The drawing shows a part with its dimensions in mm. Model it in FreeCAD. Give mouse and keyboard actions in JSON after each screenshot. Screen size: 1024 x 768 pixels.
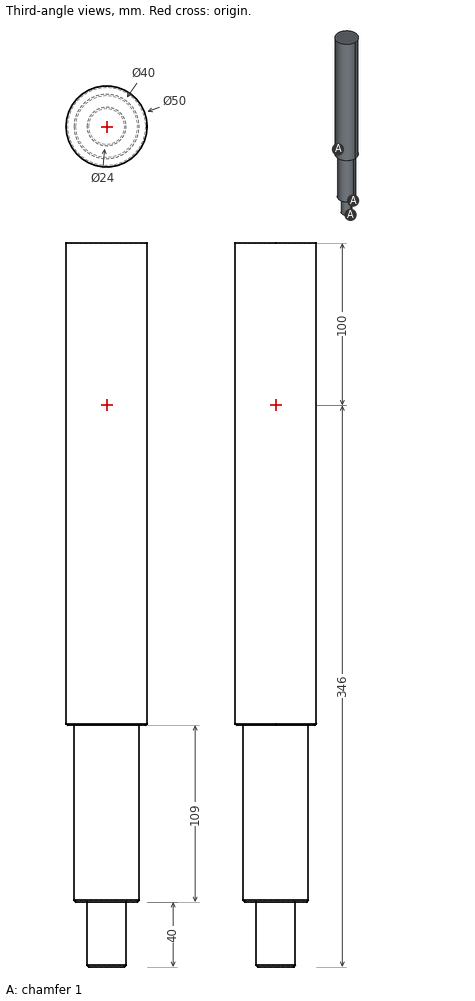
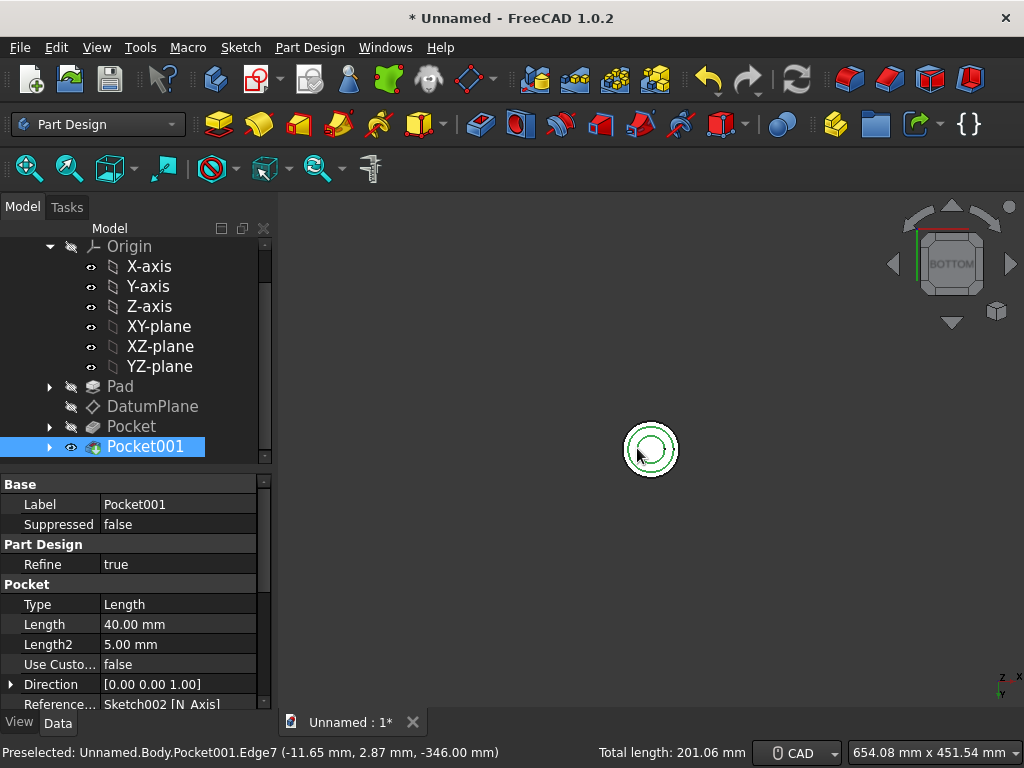
{"action": "left_click", "coordinate": [622, 448], "text": "ctrl"}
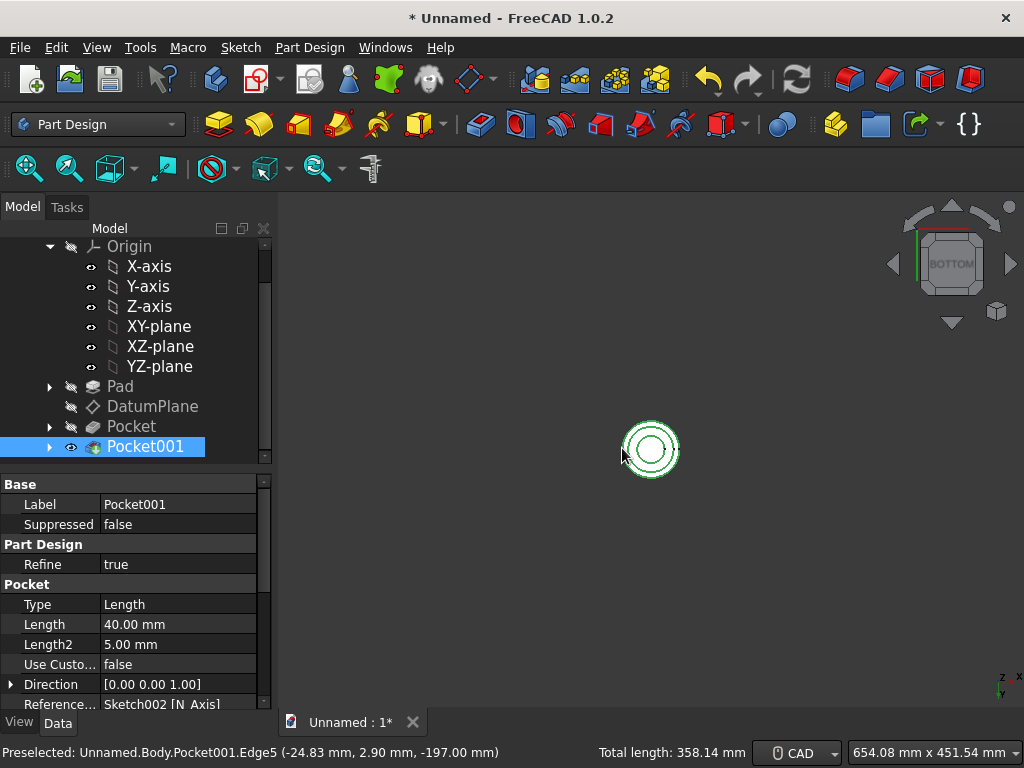
{"action": "left_click", "coordinate": [890, 80]}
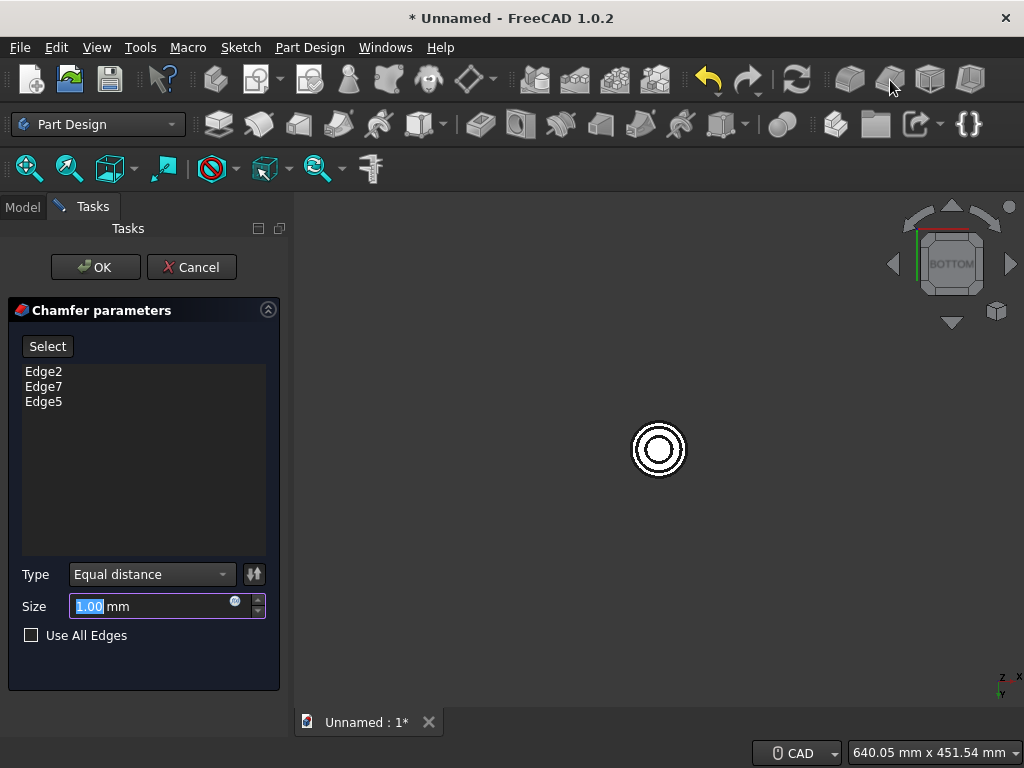
{"action": "type", "text": "1"}
{"action": "key", "text": "Tab"}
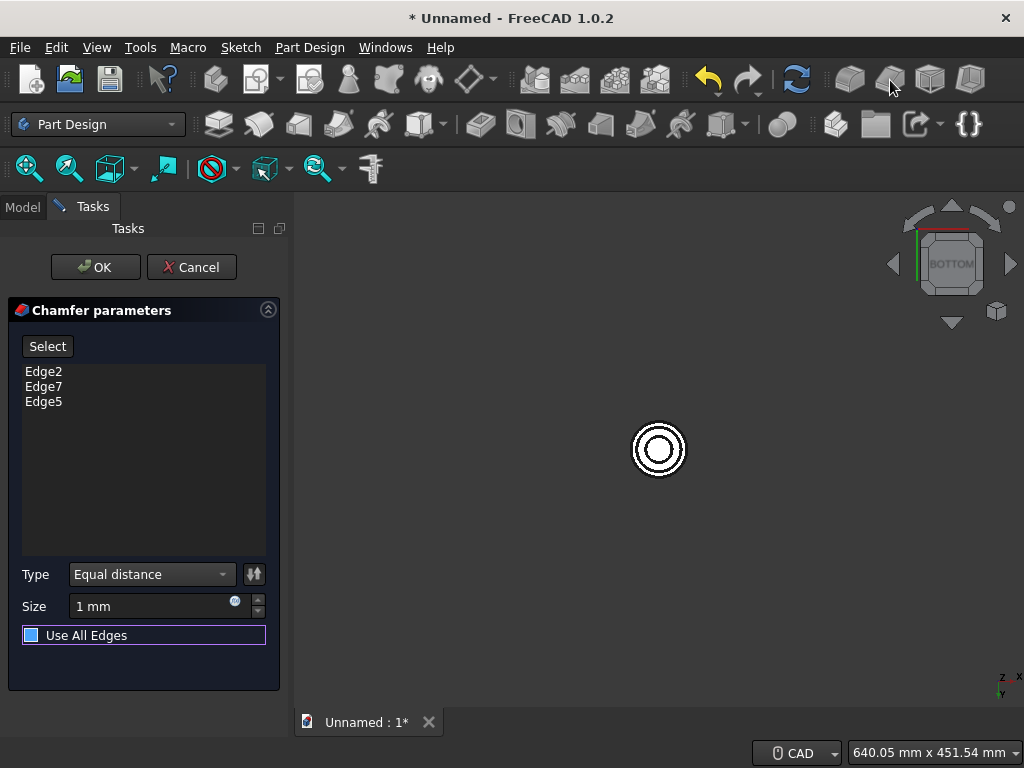
{"action": "left_click", "coordinate": [96, 267]}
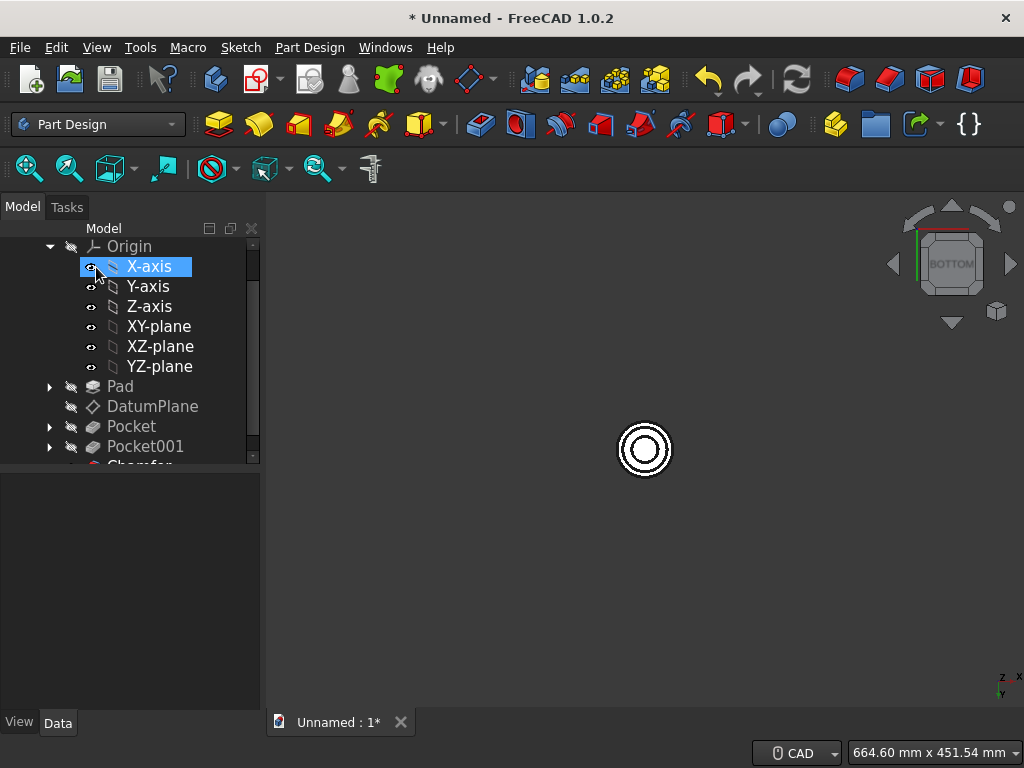
{"action": "key", "text": "0"}